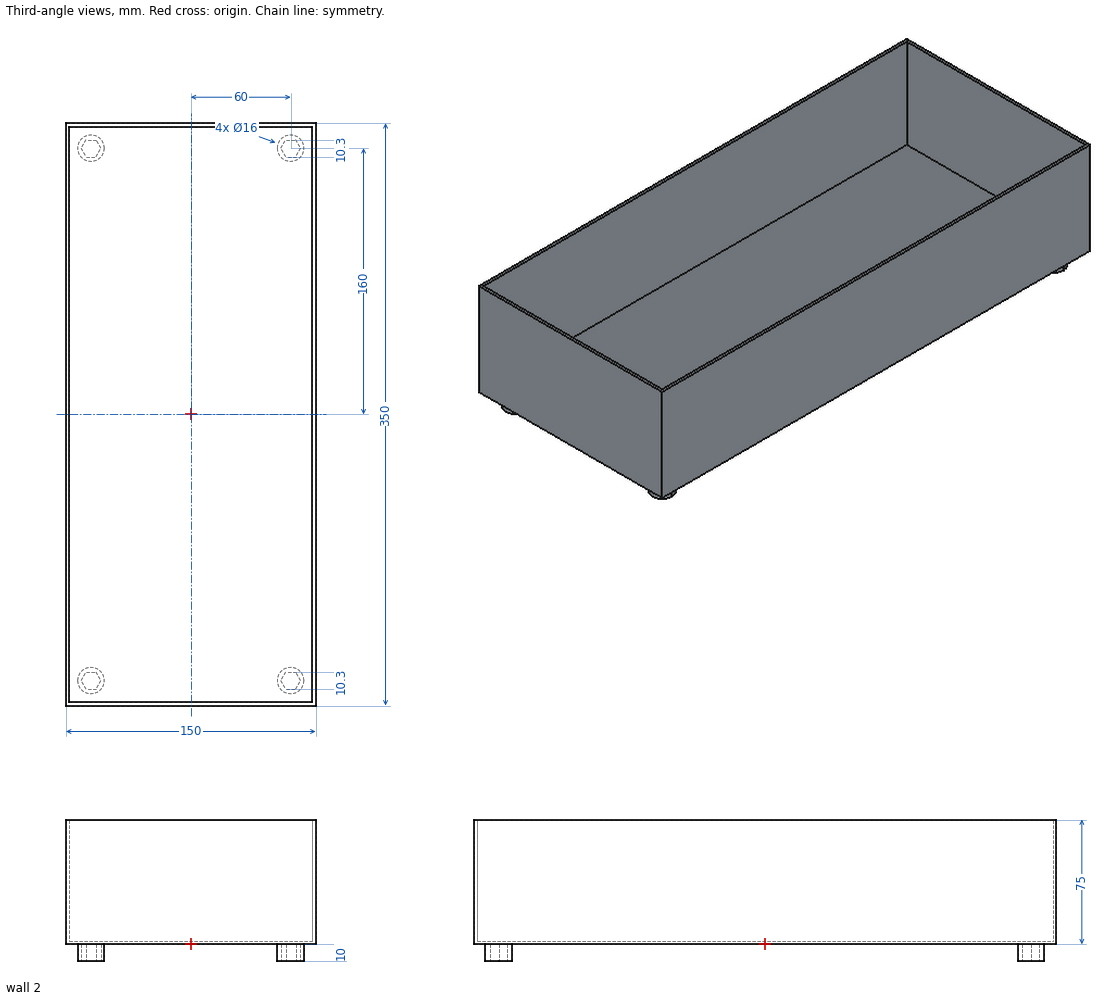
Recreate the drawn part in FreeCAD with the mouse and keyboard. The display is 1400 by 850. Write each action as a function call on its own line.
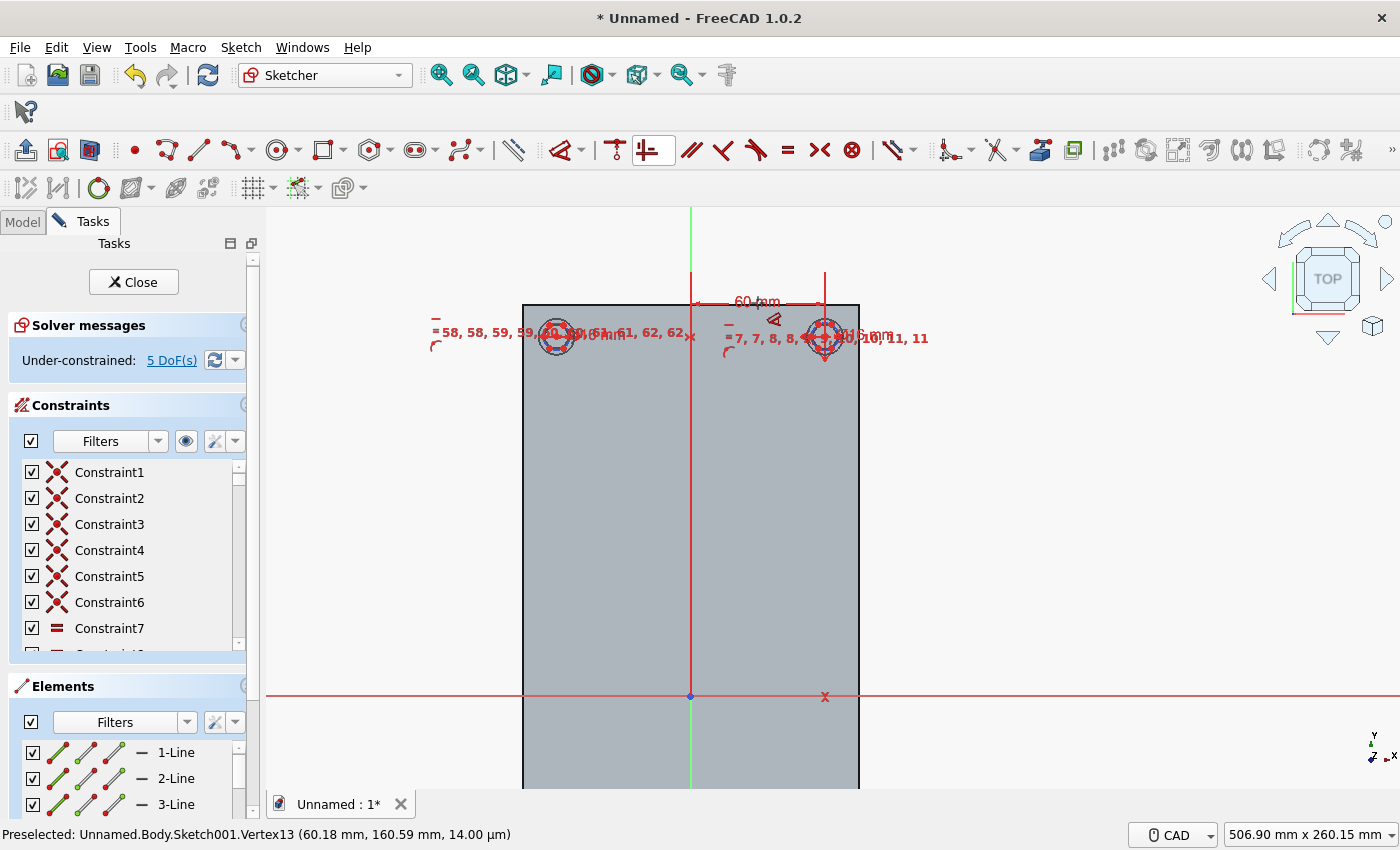
scroll(818, 349, up, 3)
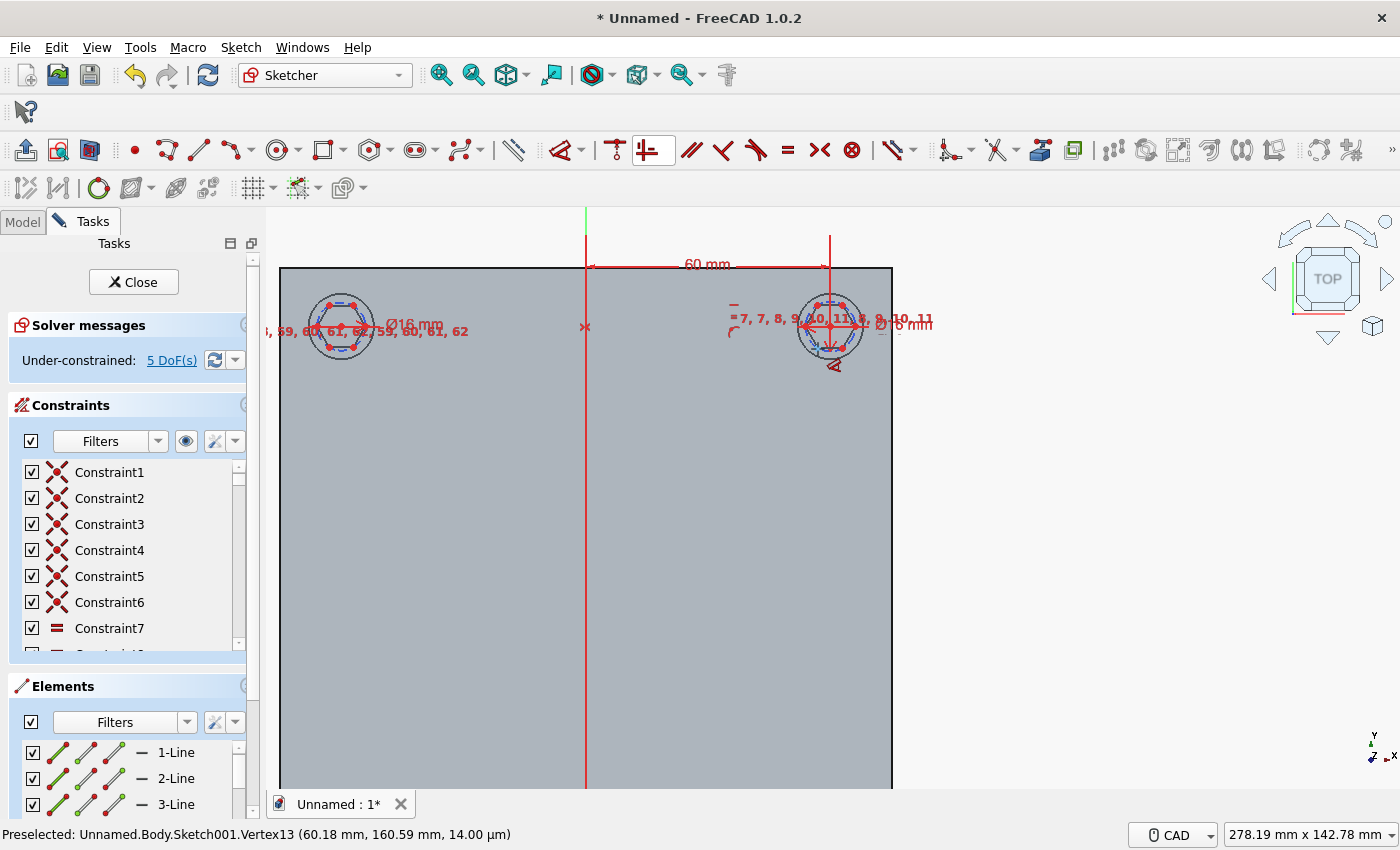
click(818, 348)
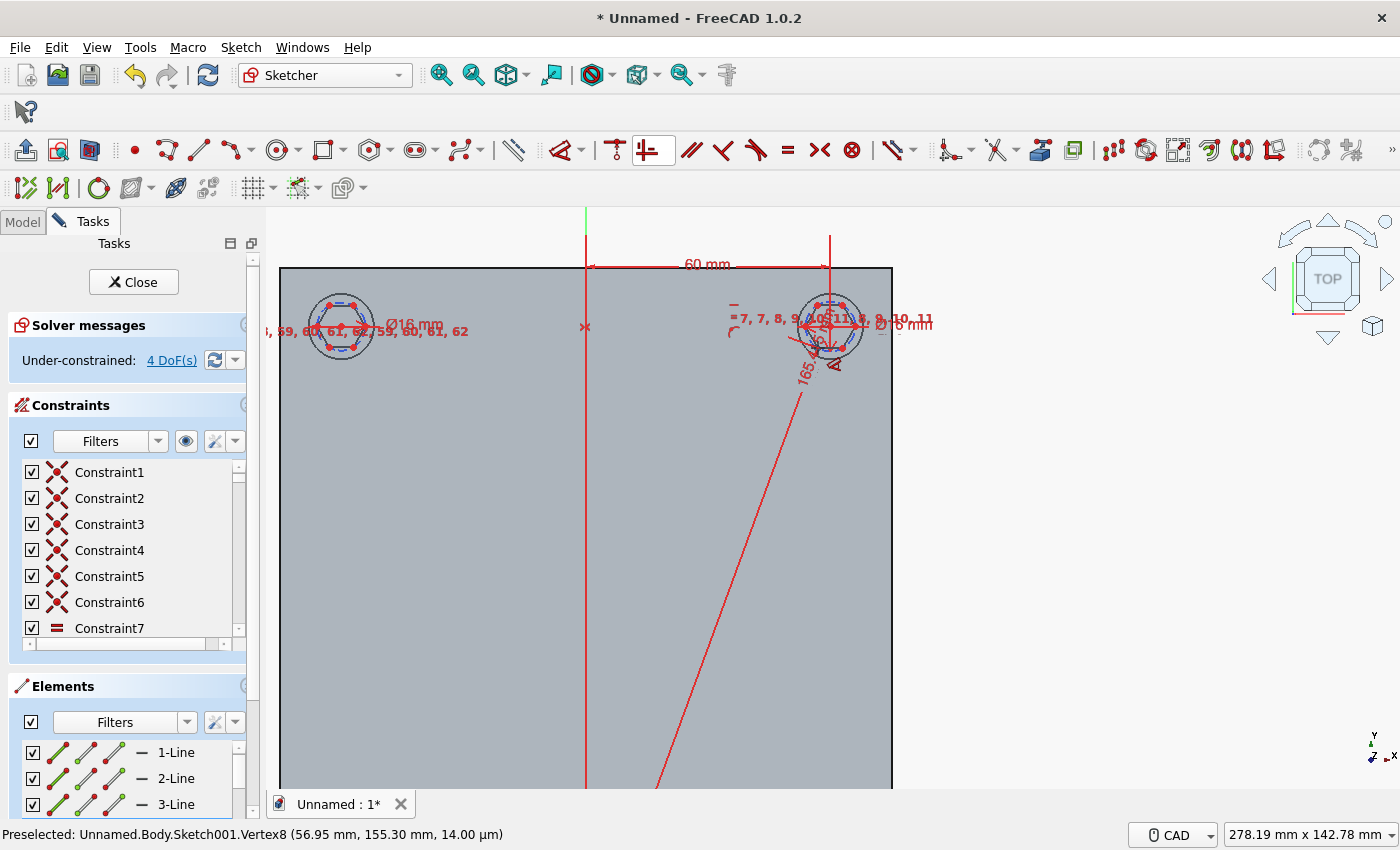
click(843, 305)
click(877, 327)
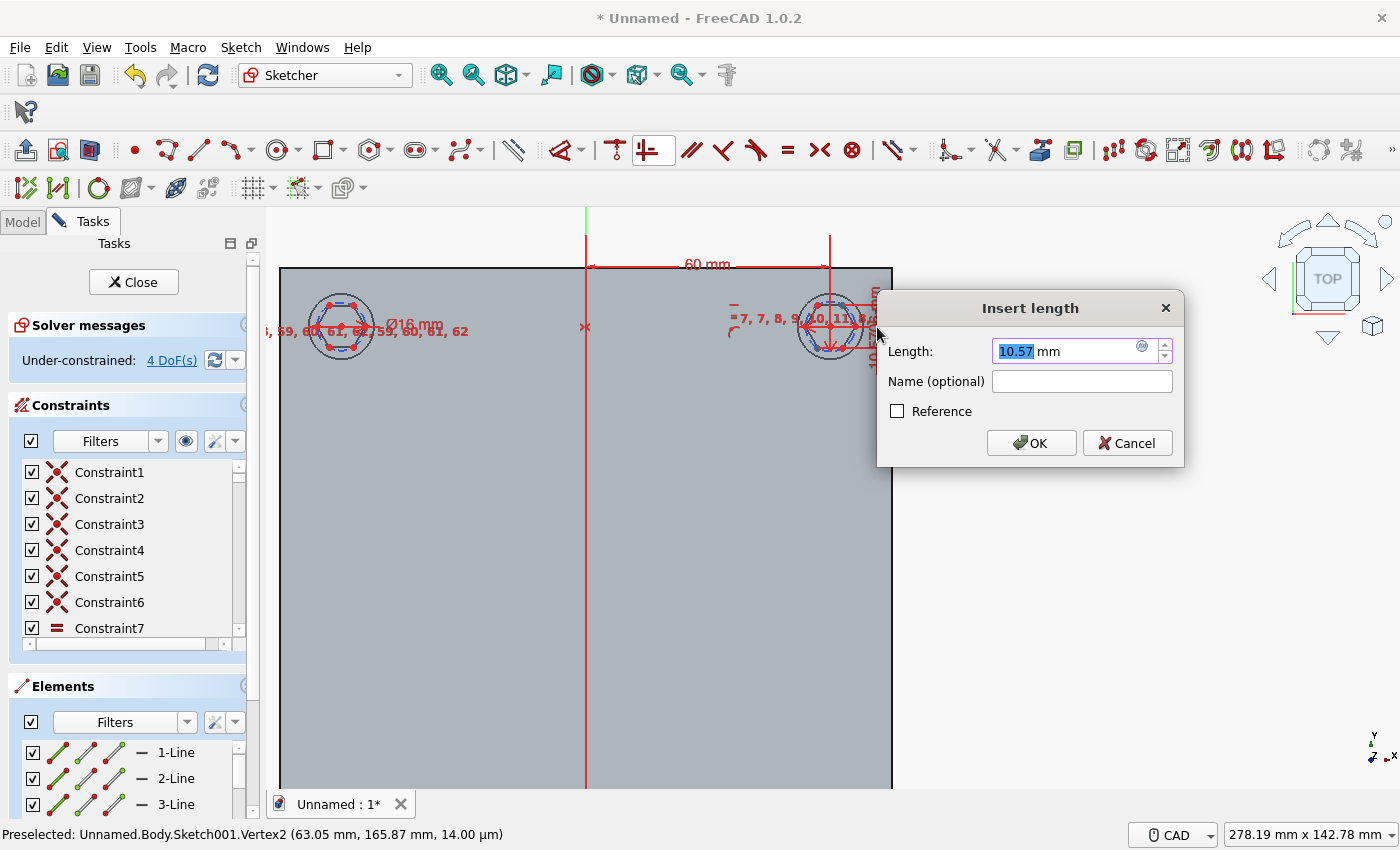
text(10.3)
key(Return)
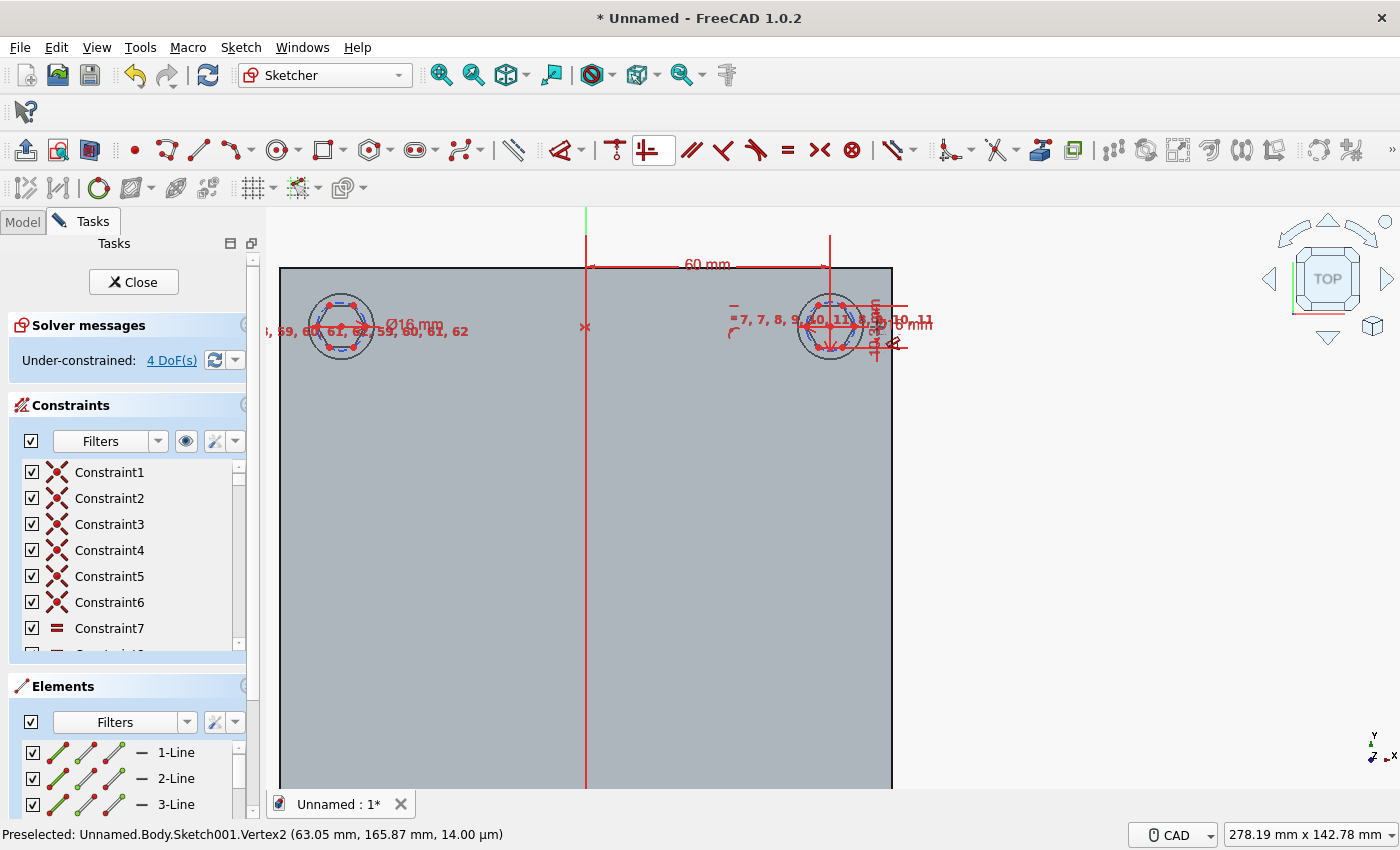
scroll(823, 340, down, 7)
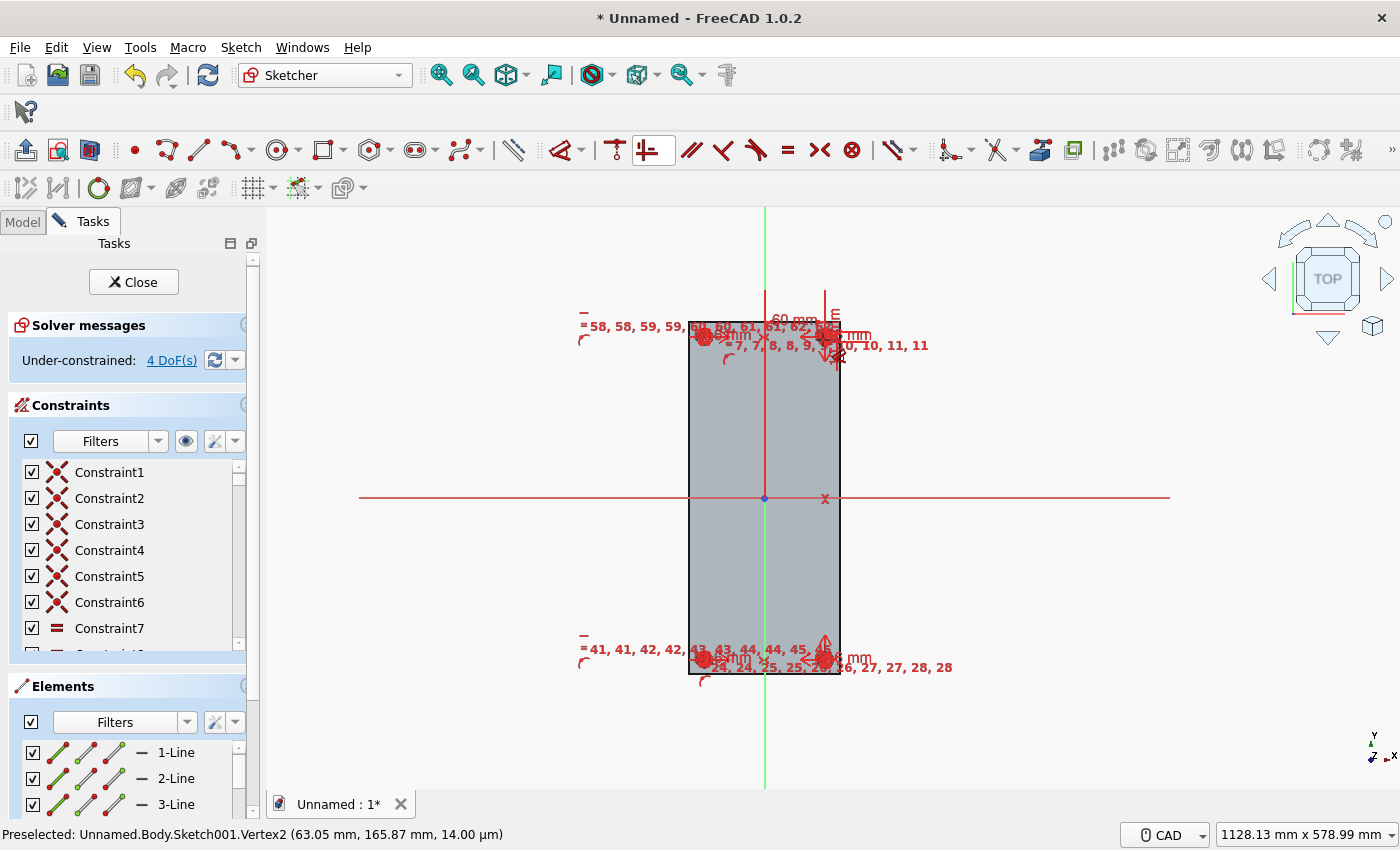
scroll(822, 665, up, 7)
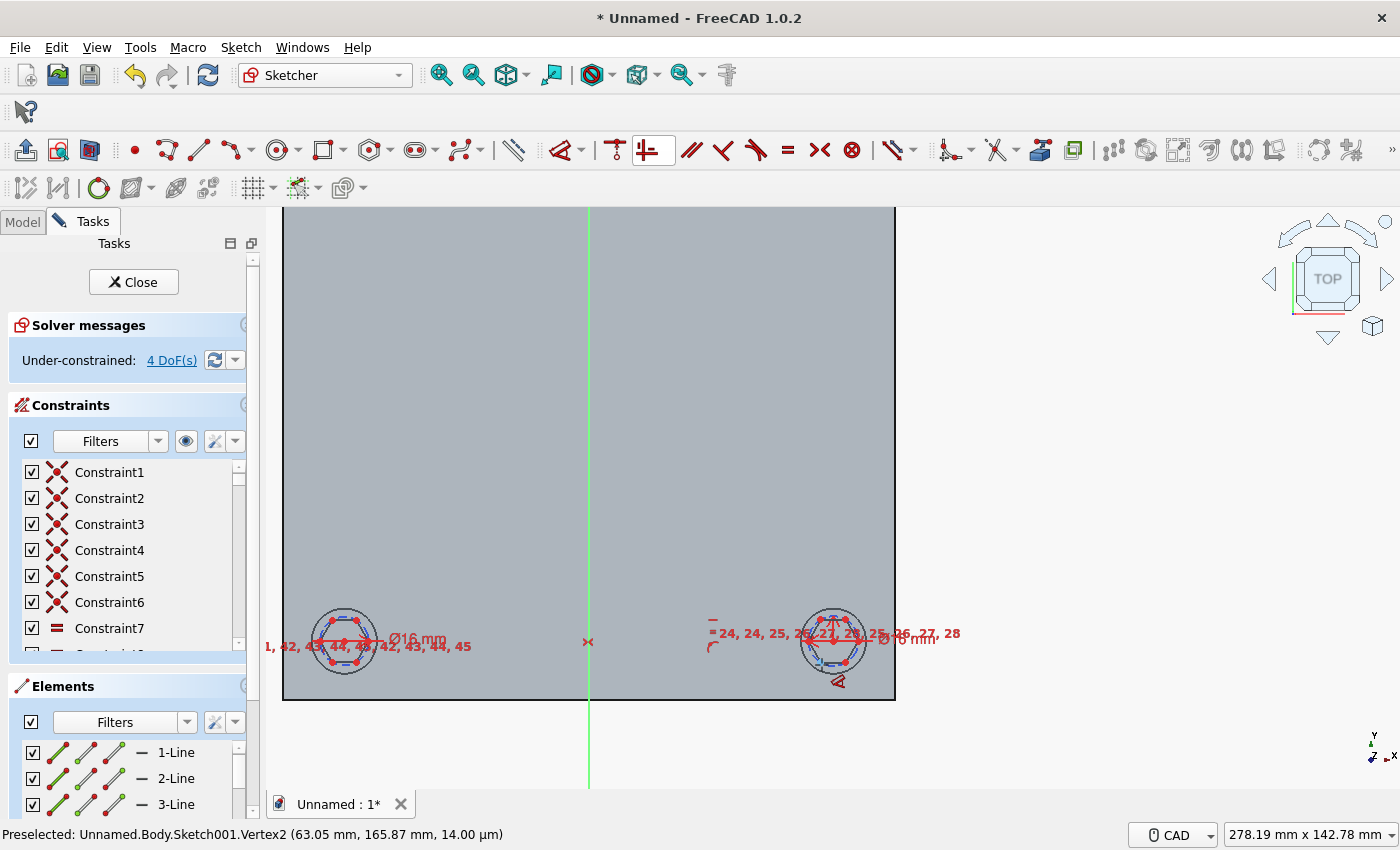
click(821, 663)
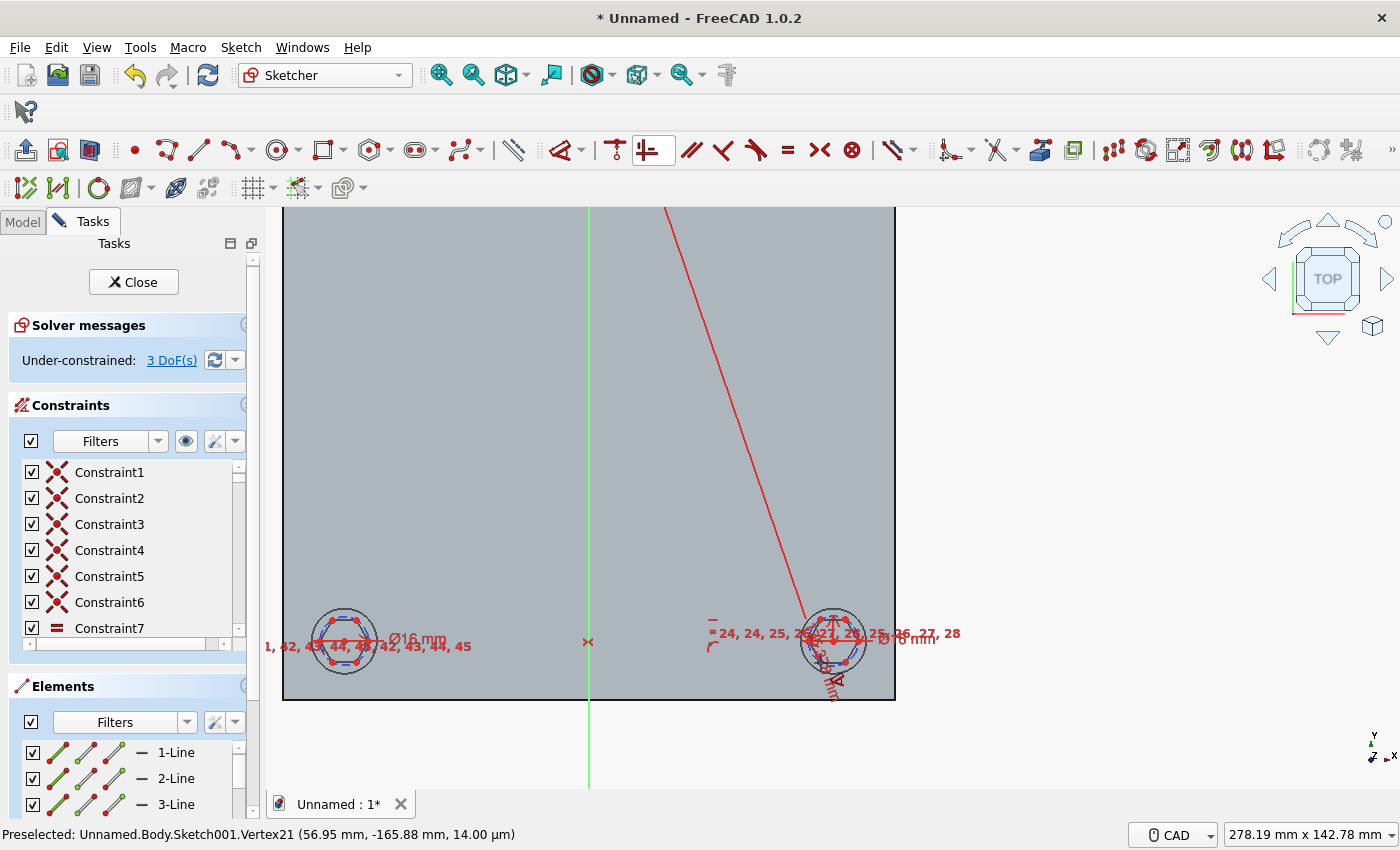
click(846, 620)
click(880, 641)